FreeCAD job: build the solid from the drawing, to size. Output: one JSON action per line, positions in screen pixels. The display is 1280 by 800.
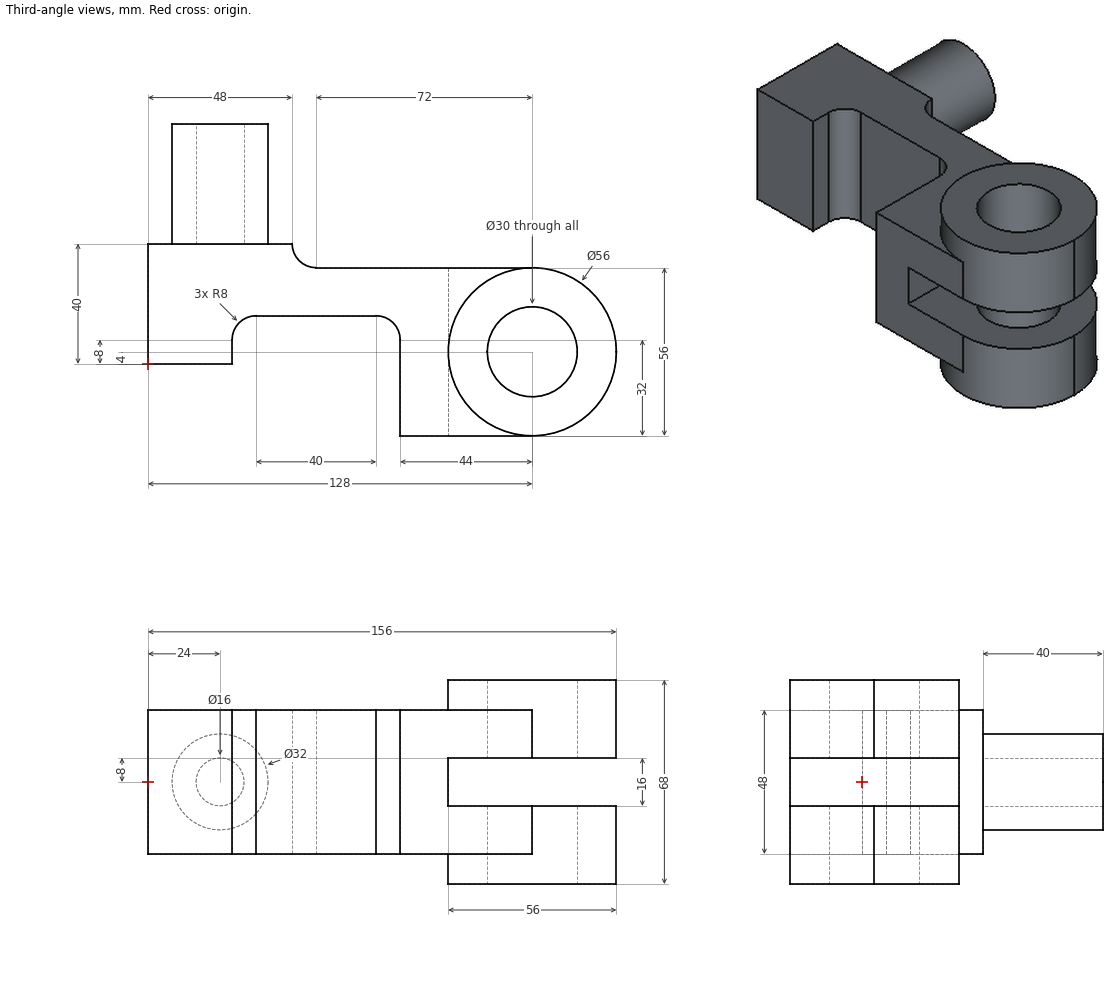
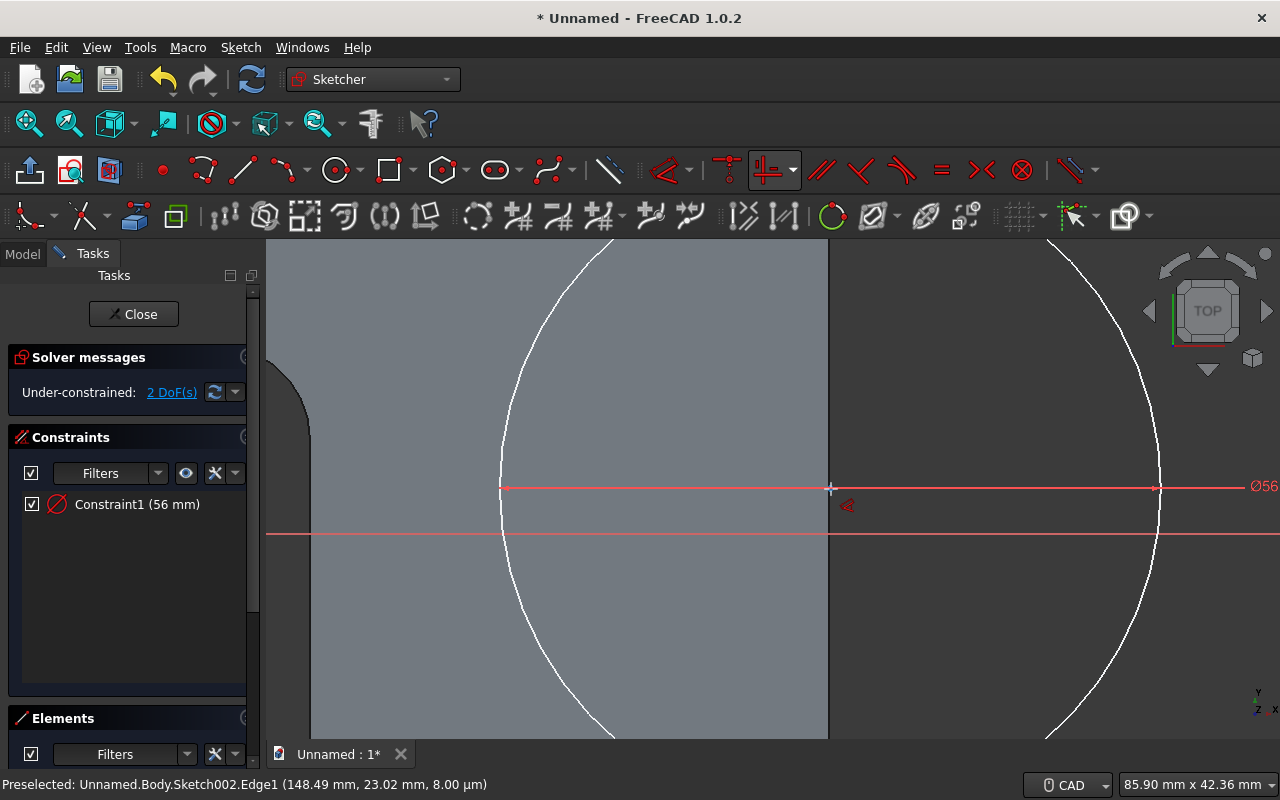
{"action": "left_click", "coordinate": [830, 488]}
{"action": "left_click", "coordinate": [864, 511]}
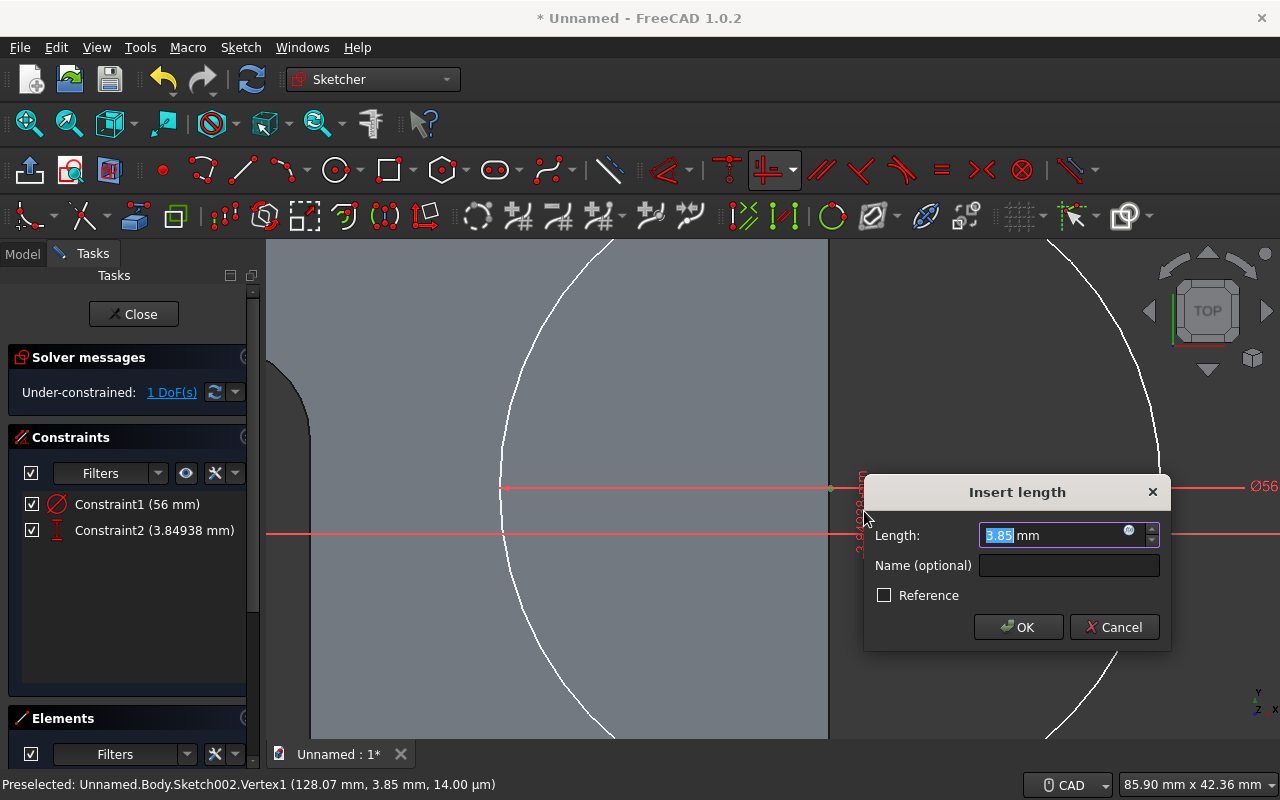
{"action": "type", "text": "4"}
{"action": "key", "text": "Return"}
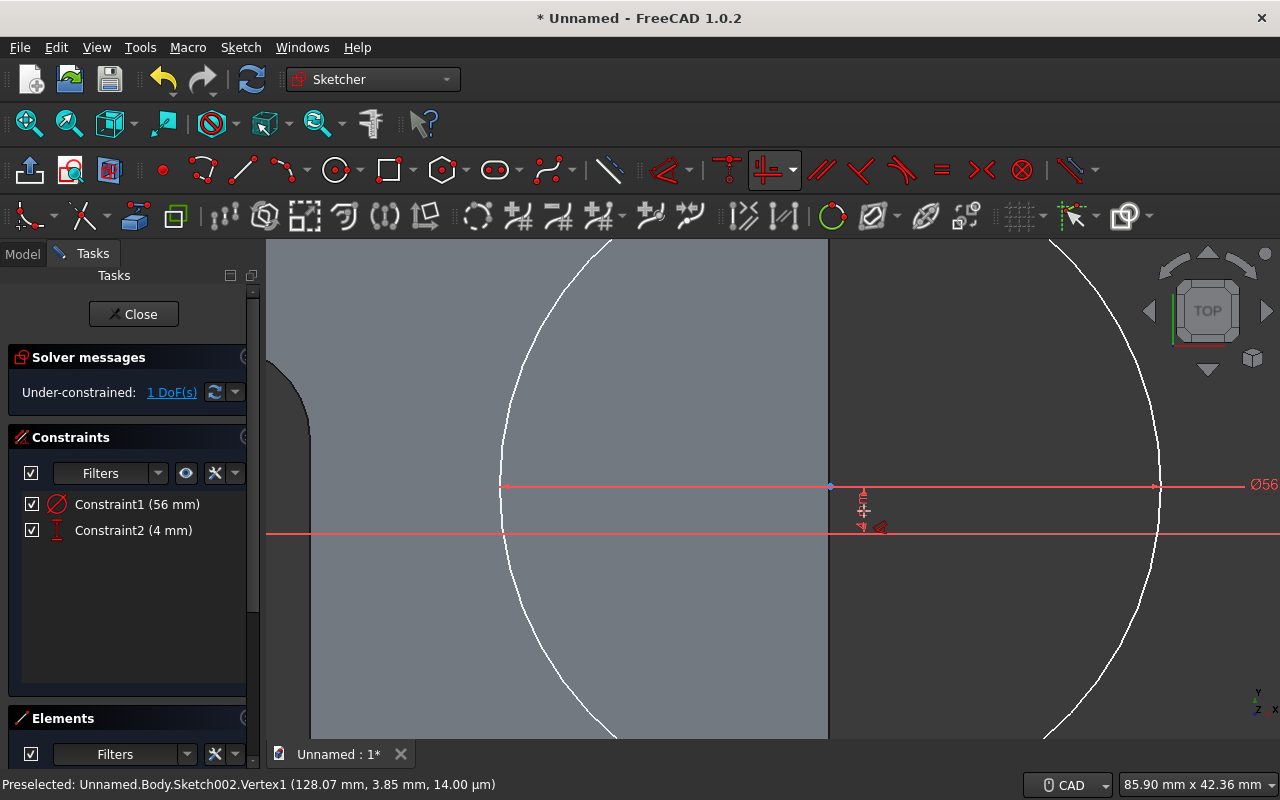
{"action": "left_click", "coordinate": [830, 487]}
{"action": "left_click", "coordinate": [562, 568]}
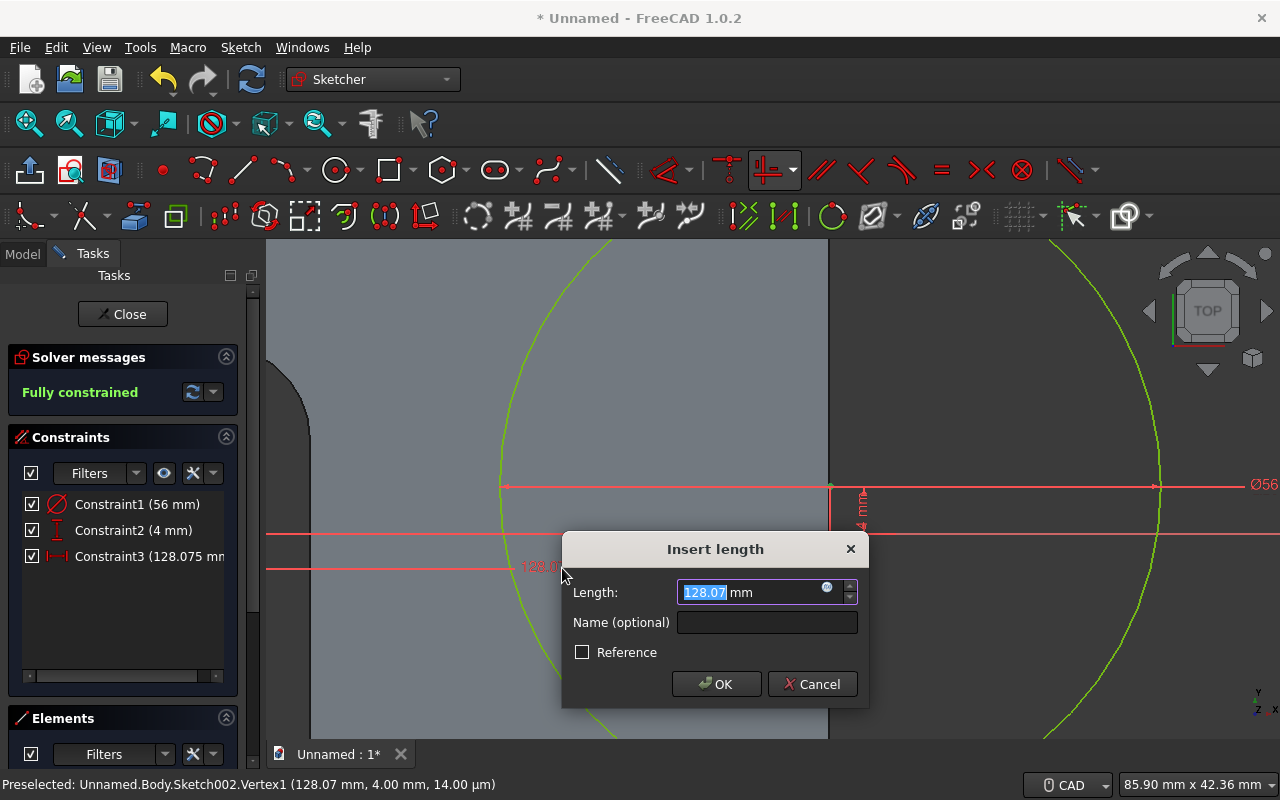
{"action": "type", "text": "128"}
{"action": "key", "text": "Return"}
{"action": "key", "text": "Escape"}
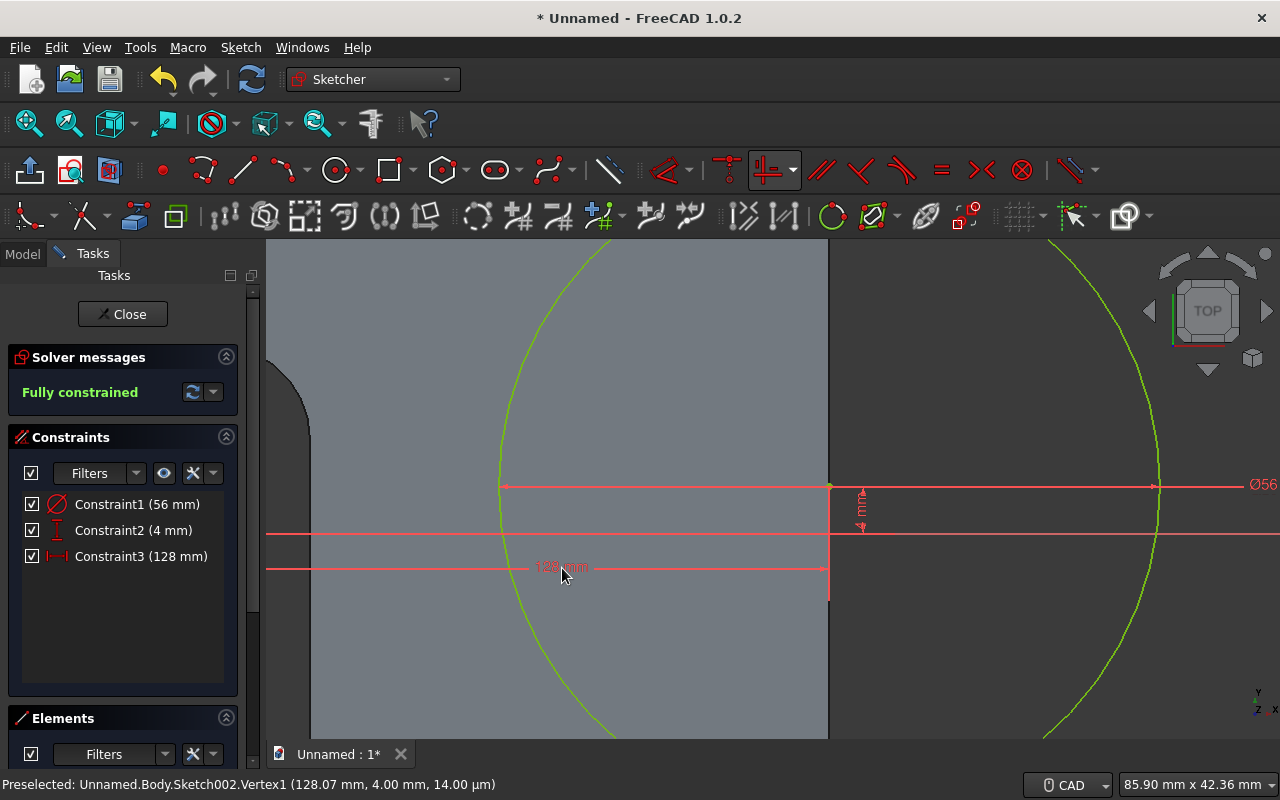
{"action": "left_click", "coordinate": [123, 314]}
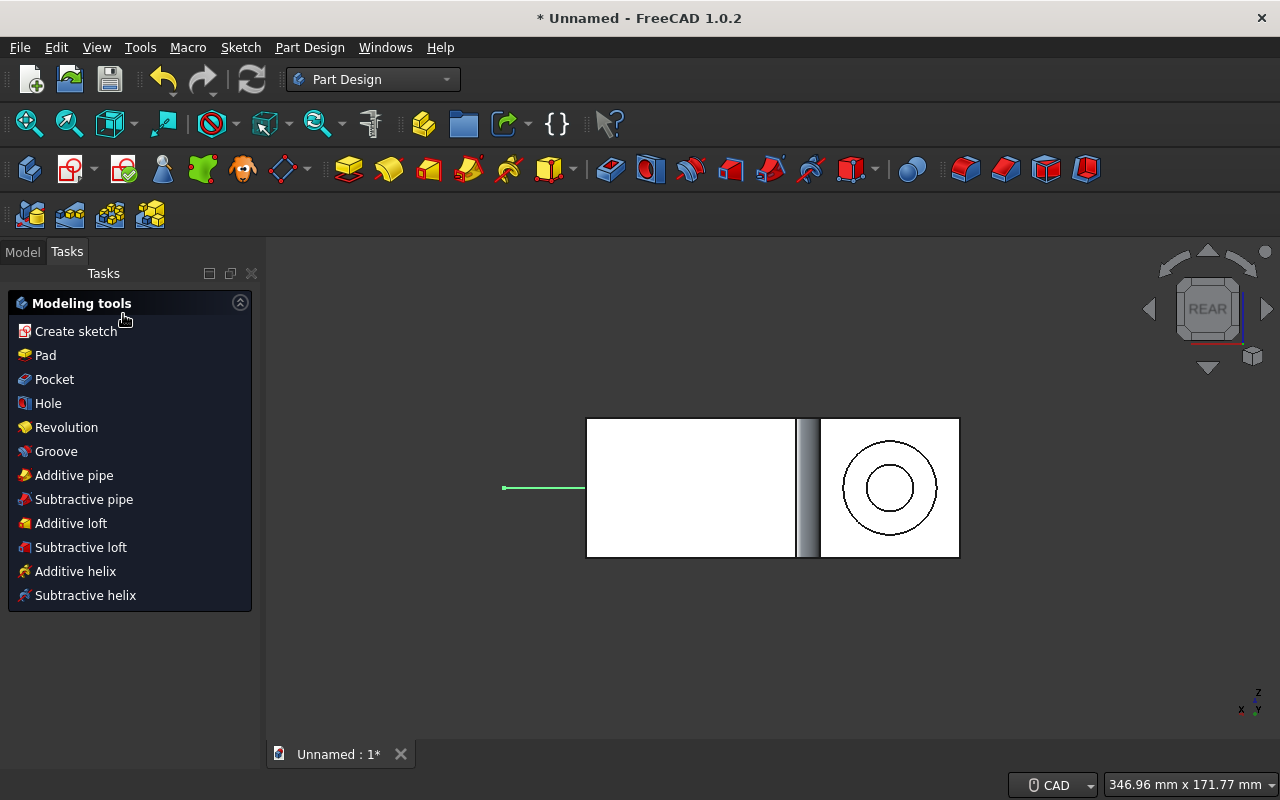
{"action": "left_click", "coordinate": [350, 170]}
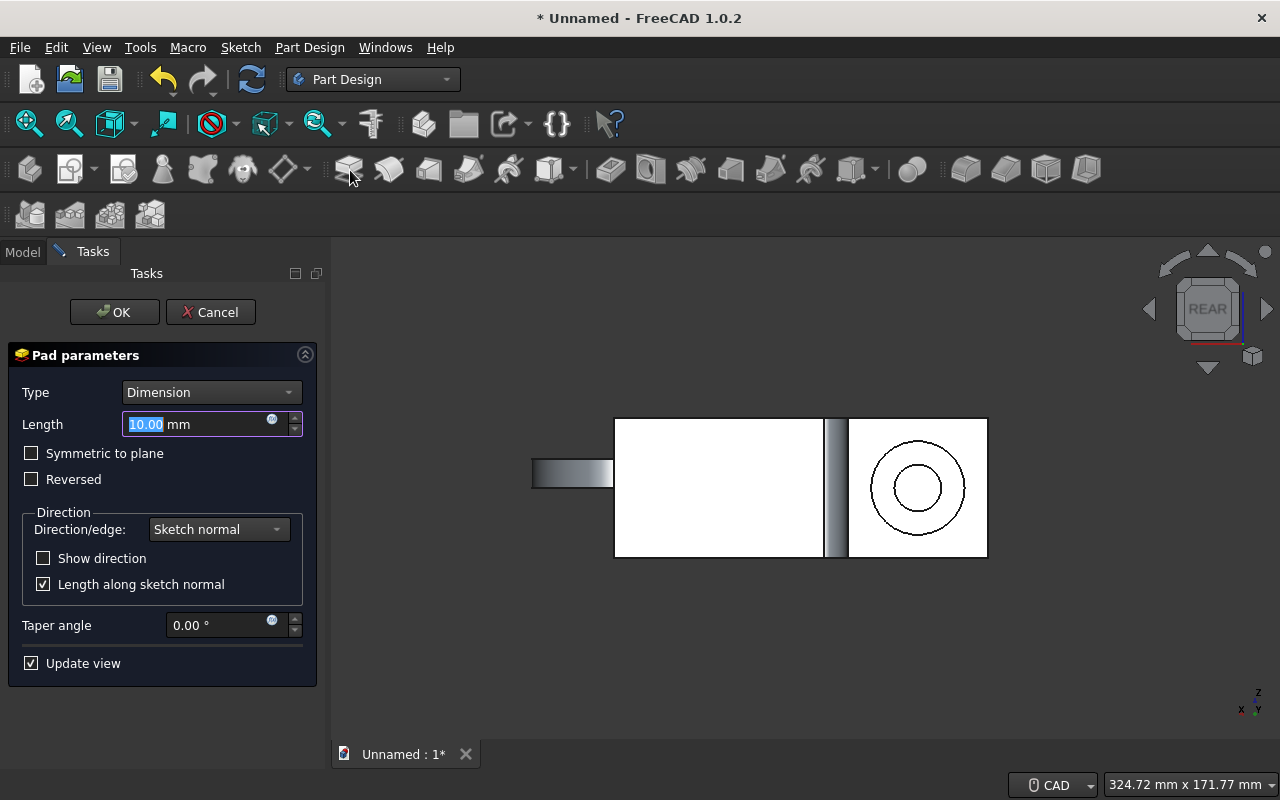
{"action": "type", "text": "68"}
{"action": "key", "text": "Tab"}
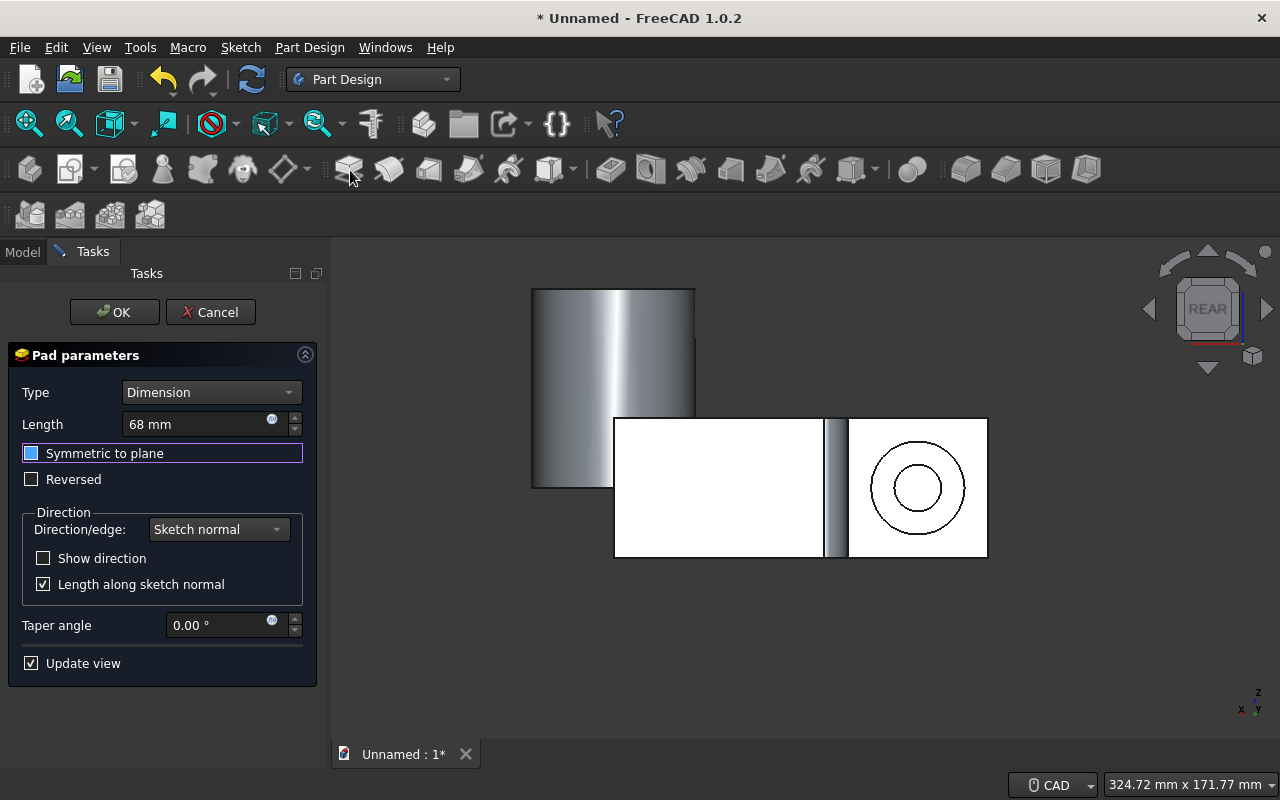
{"action": "left_click", "coordinate": [30, 453]}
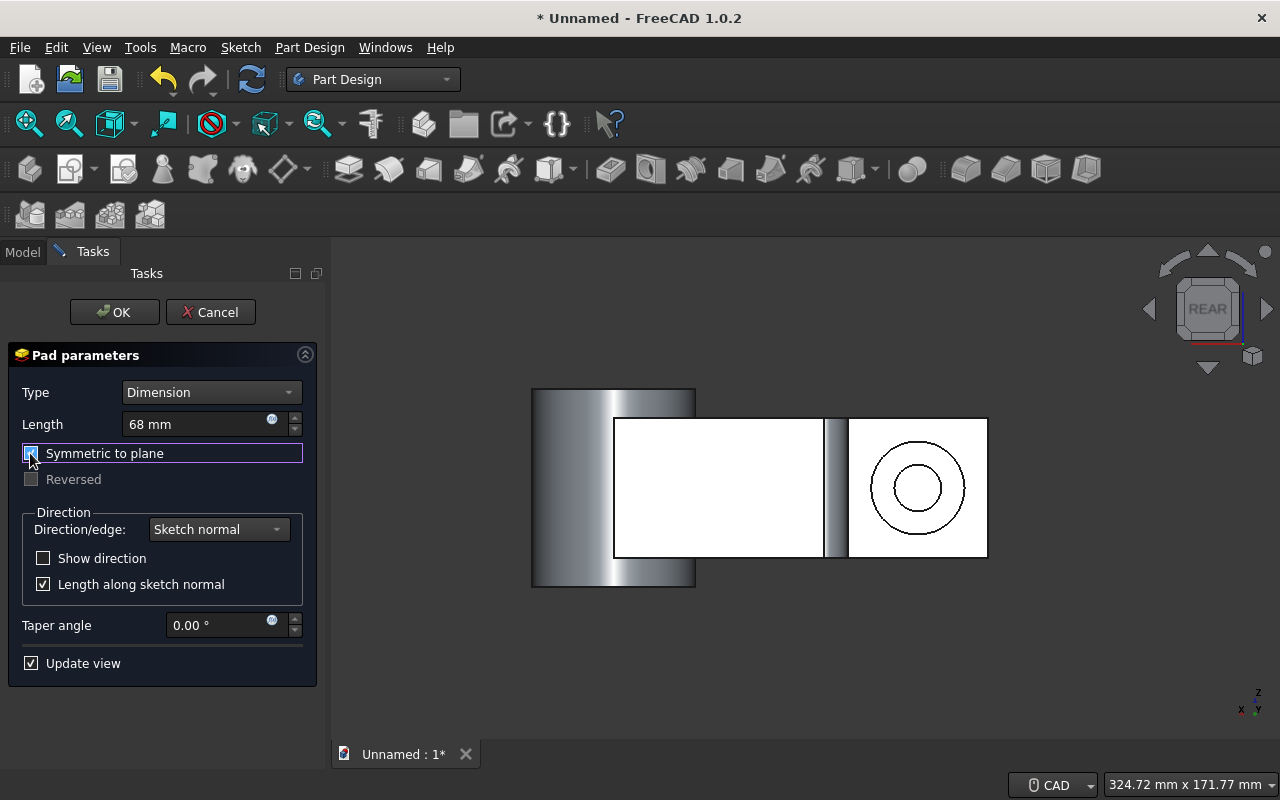
{"action": "left_click", "coordinate": [115, 312]}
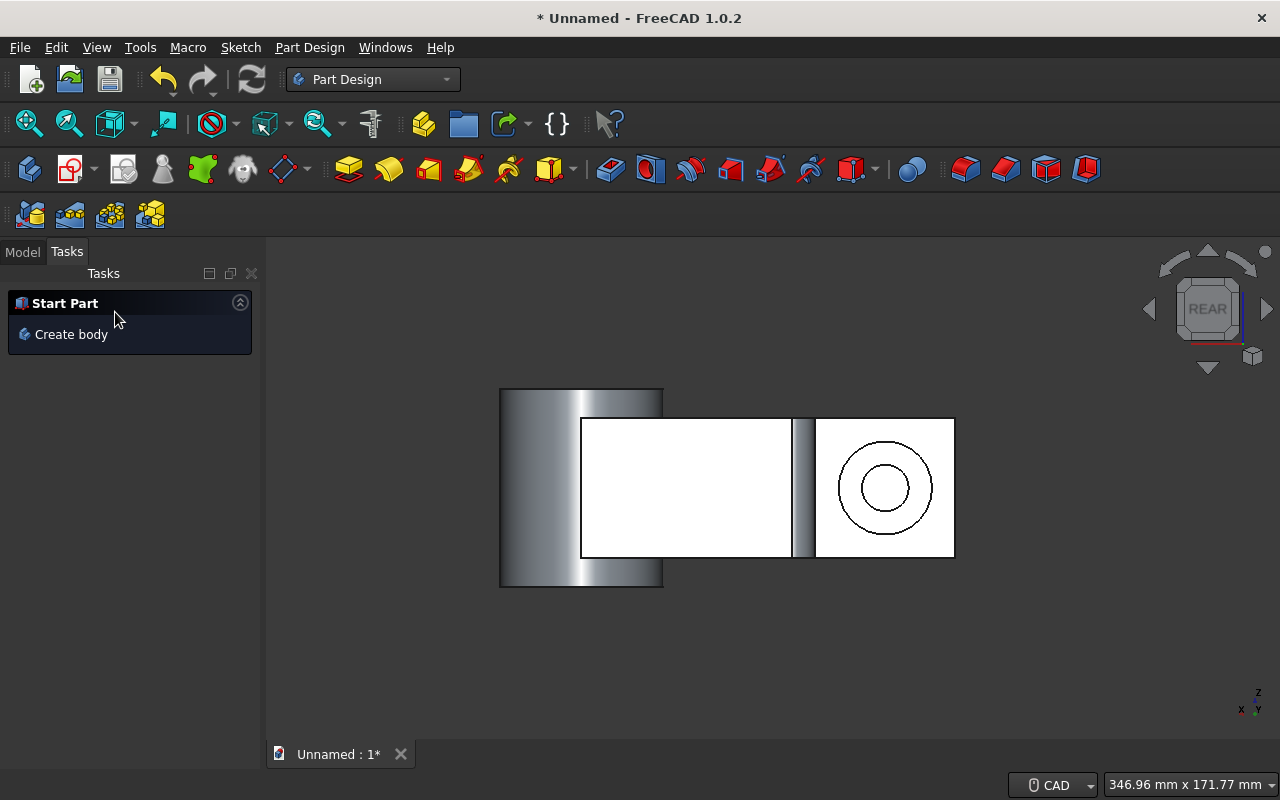
{"action": "left_click", "coordinate": [30, 124]}